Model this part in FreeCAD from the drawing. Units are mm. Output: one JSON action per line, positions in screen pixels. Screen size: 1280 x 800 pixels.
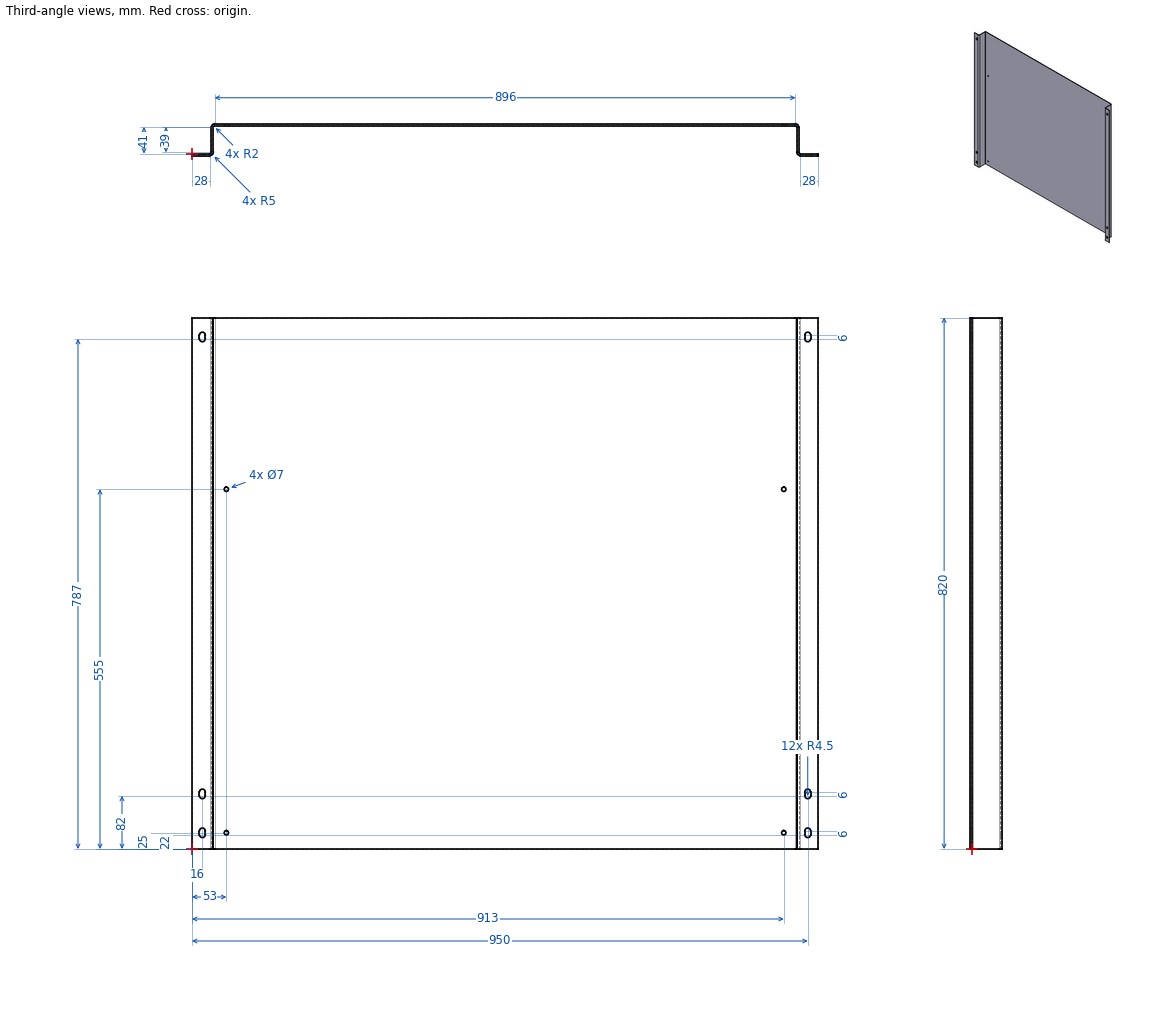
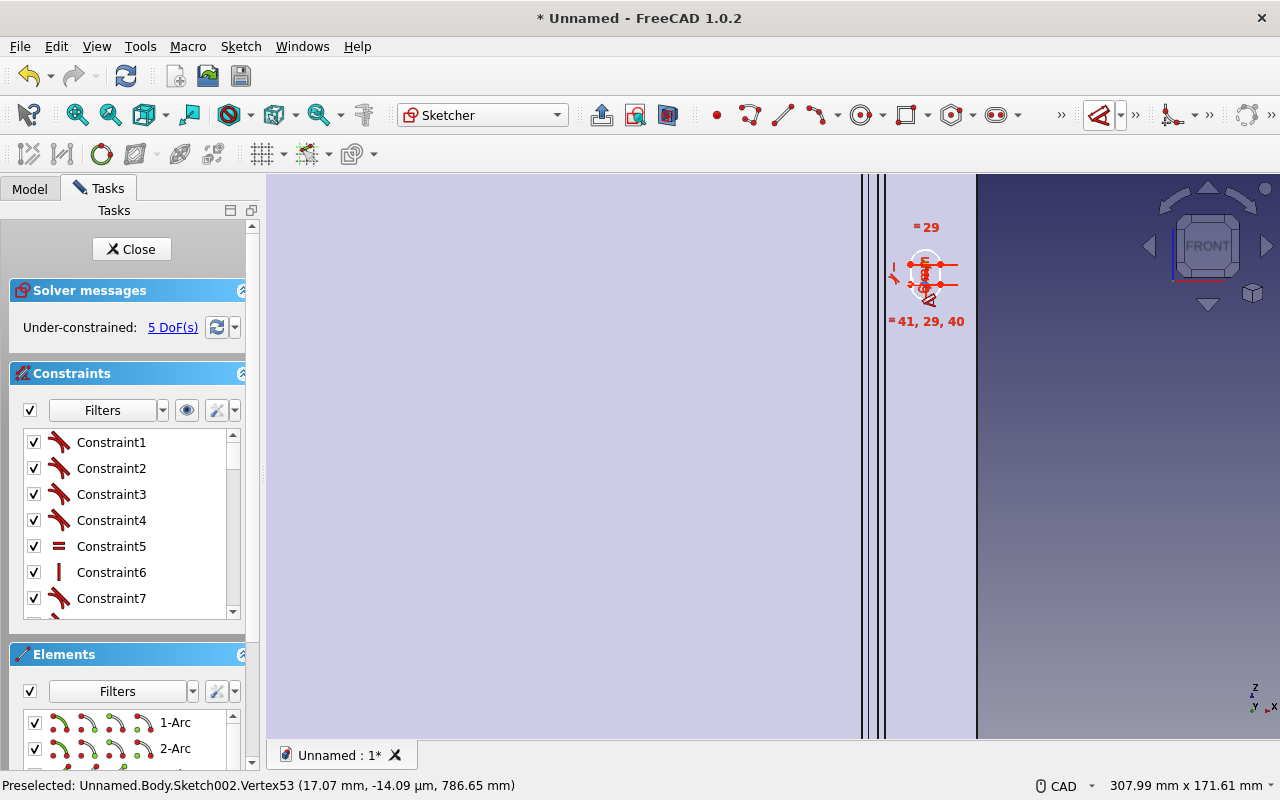
{"action": "left_click", "coordinate": [911, 285]}
{"action": "left_click", "coordinate": [945, 498]}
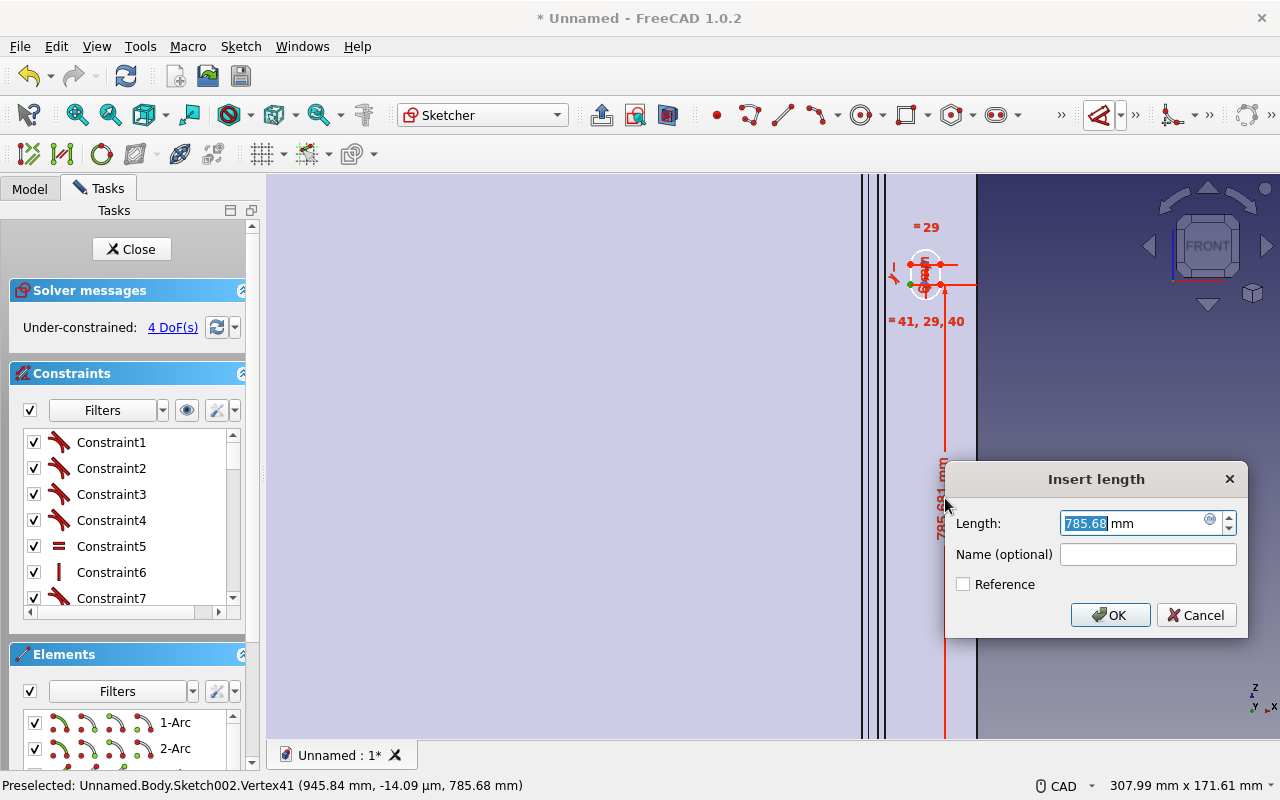
{"action": "type", "text": "787"}
{"action": "key", "text": "Return"}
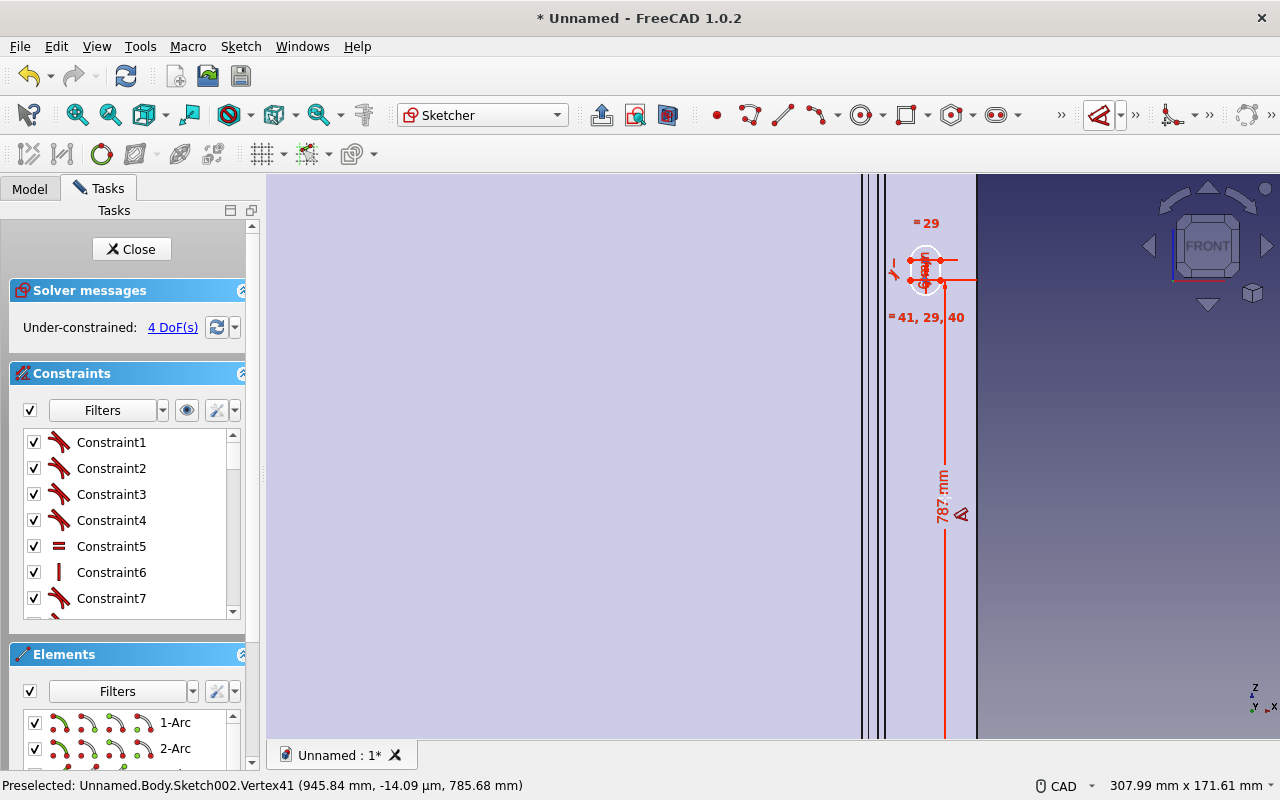
{"action": "scroll", "coordinate": [914, 284], "scroll_direction": "down", "scroll_amount": 10}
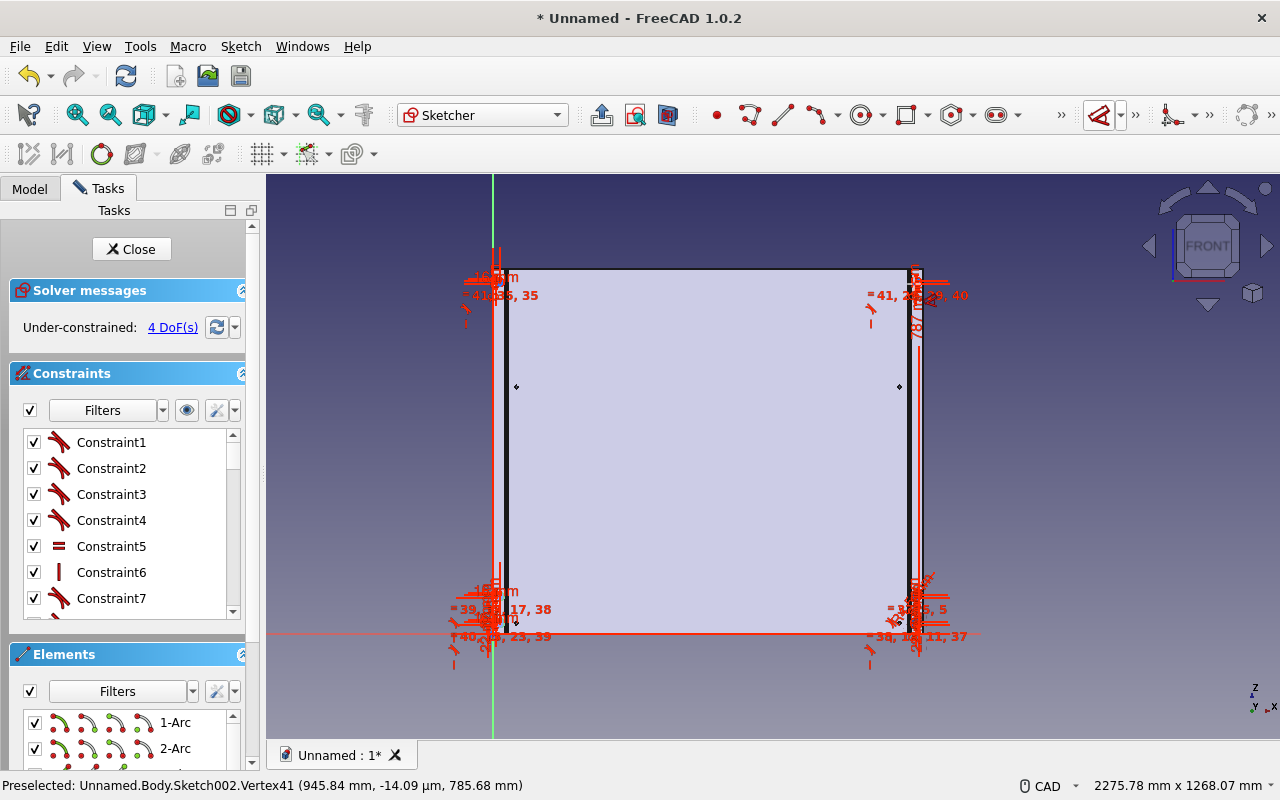
{"action": "scroll", "coordinate": [498, 284], "scroll_direction": "up", "scroll_amount": 10}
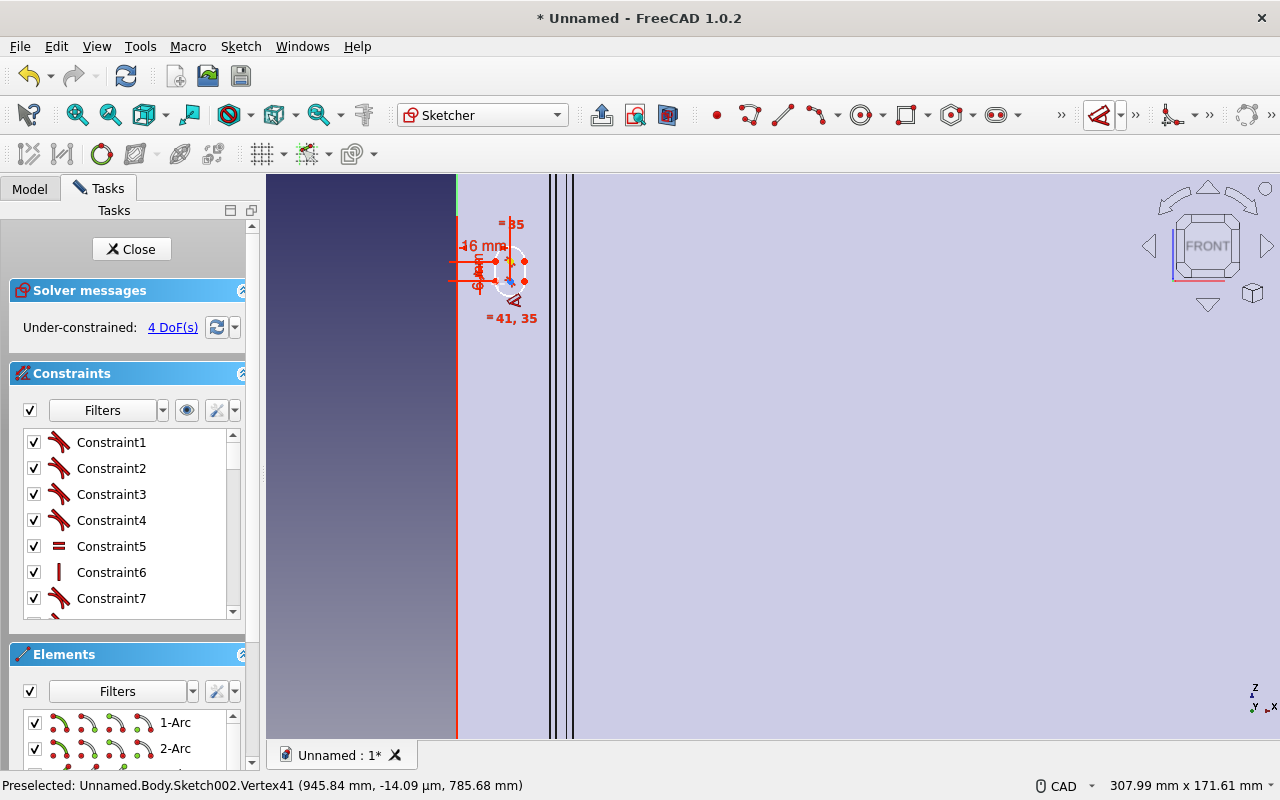
{"action": "left_click", "coordinate": [495, 281]}
{"action": "left_click", "coordinate": [423, 496]}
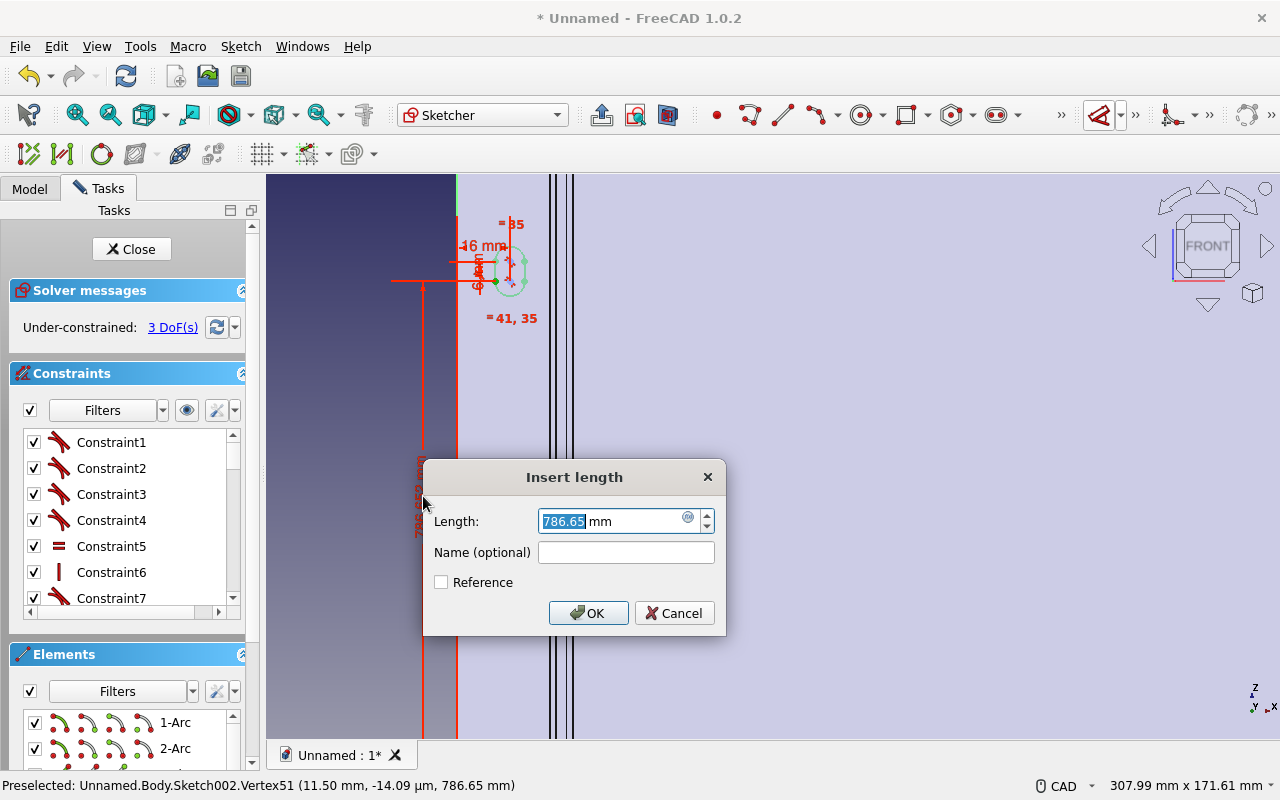
{"action": "type", "text": "787"}
{"action": "key", "text": "Return"}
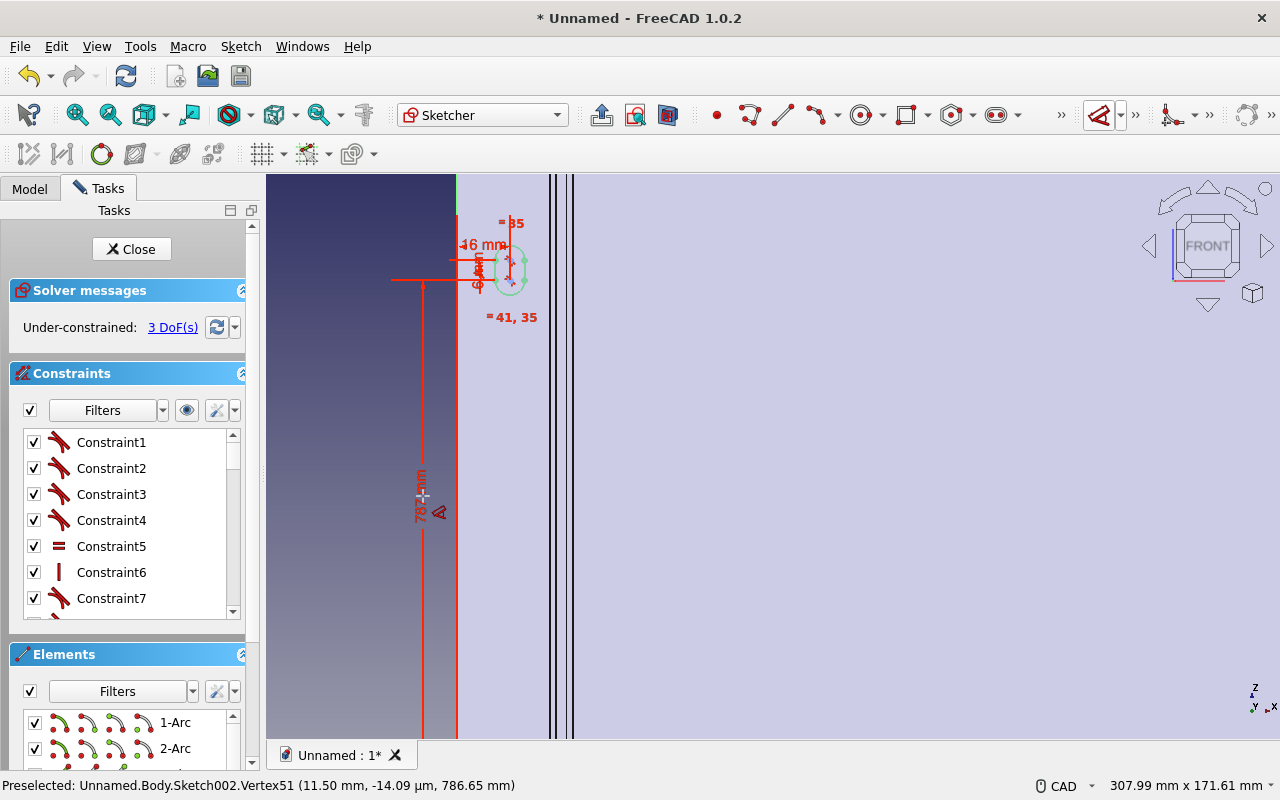
{"action": "scroll", "coordinate": [497, 284], "scroll_direction": "down", "scroll_amount": 10}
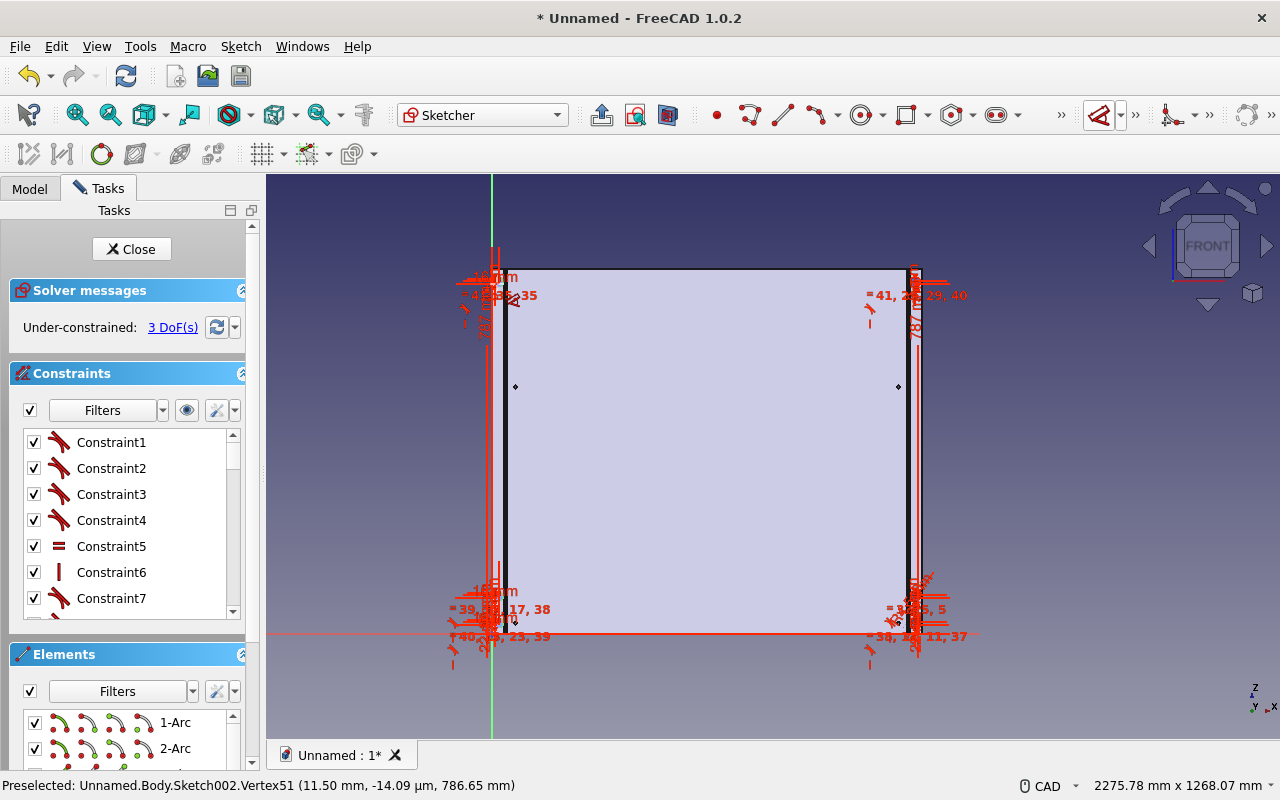
{"action": "scroll", "coordinate": [915, 598], "scroll_direction": "up", "scroll_amount": 10}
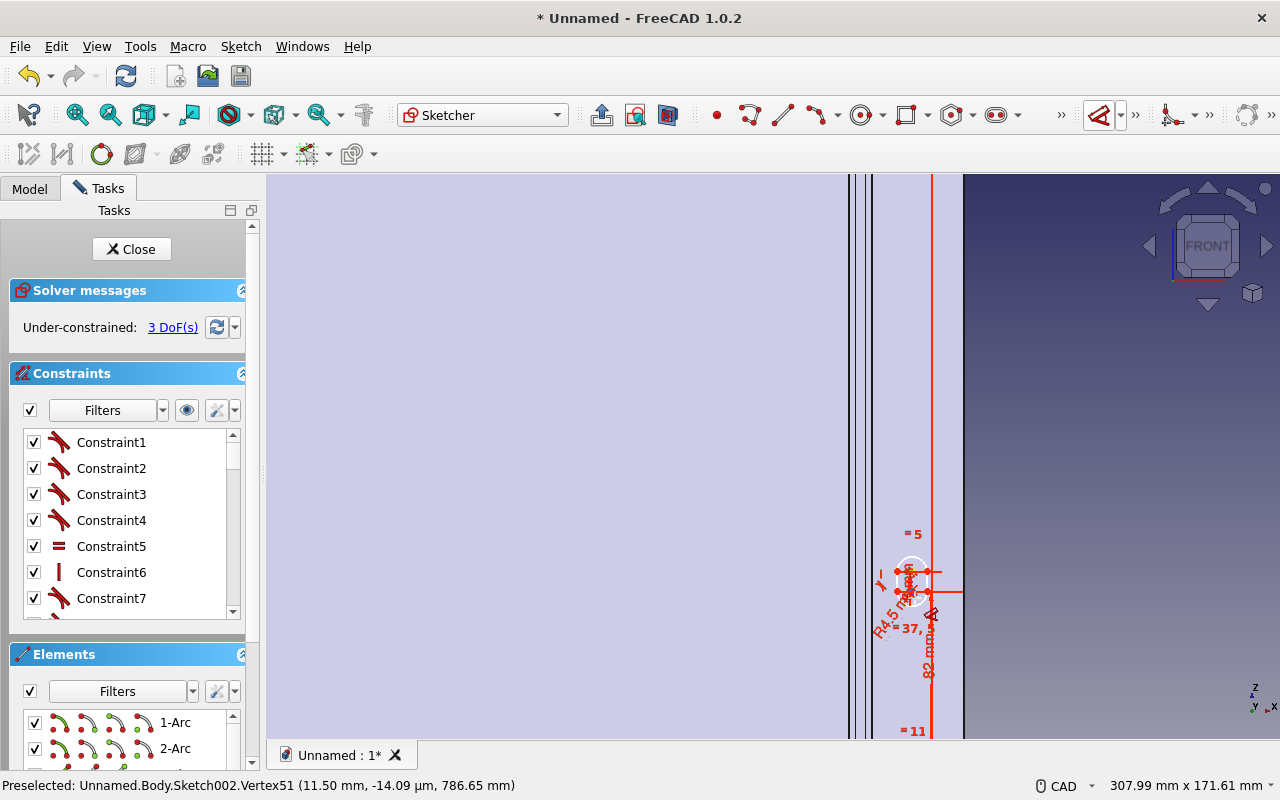
{"action": "left_click", "coordinate": [912, 592]}
{"action": "left_click", "coordinate": [603, 558]}